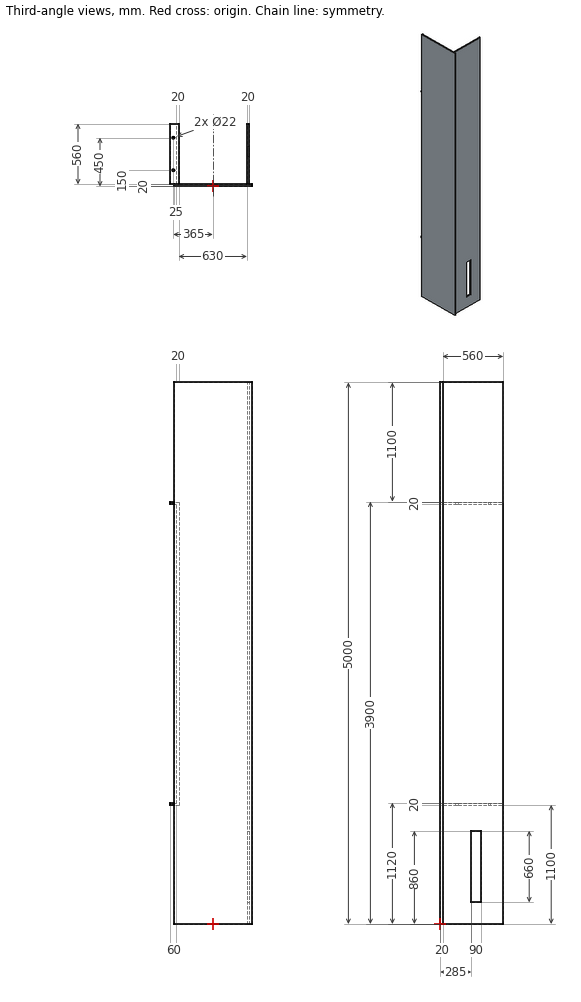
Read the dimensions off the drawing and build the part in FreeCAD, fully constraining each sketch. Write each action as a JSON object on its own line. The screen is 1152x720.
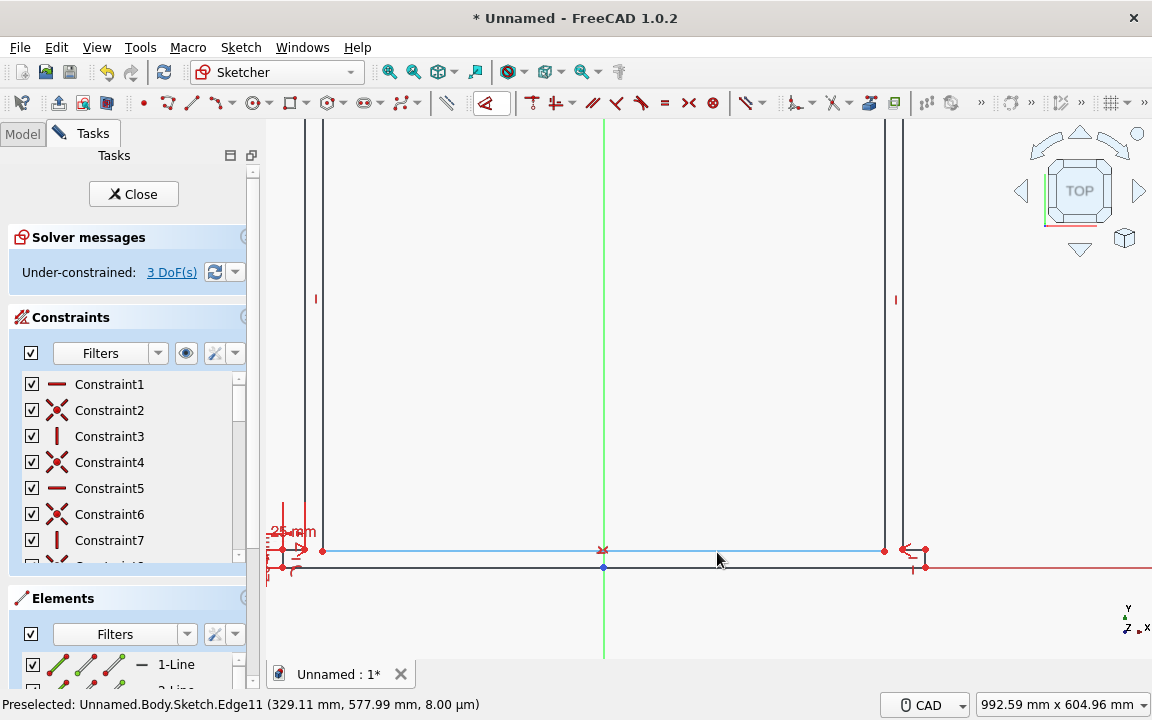
{"action": "left_click", "coordinate": [716, 551]}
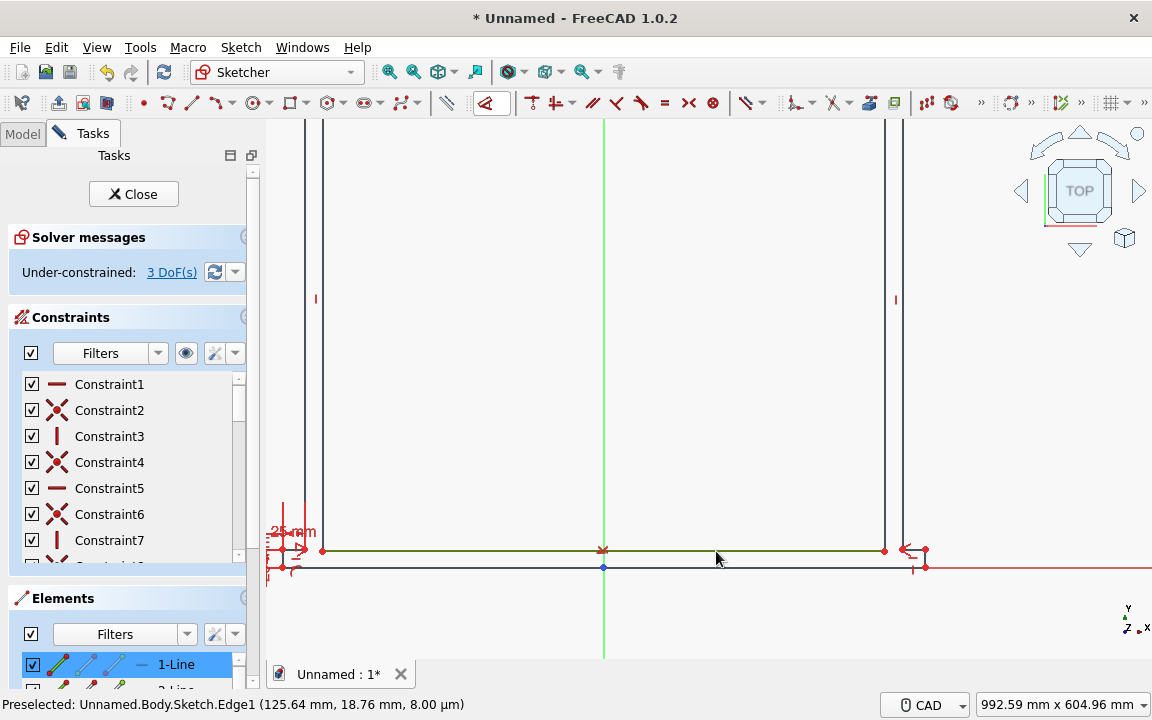
{"action": "left_click", "coordinate": [504, 104]}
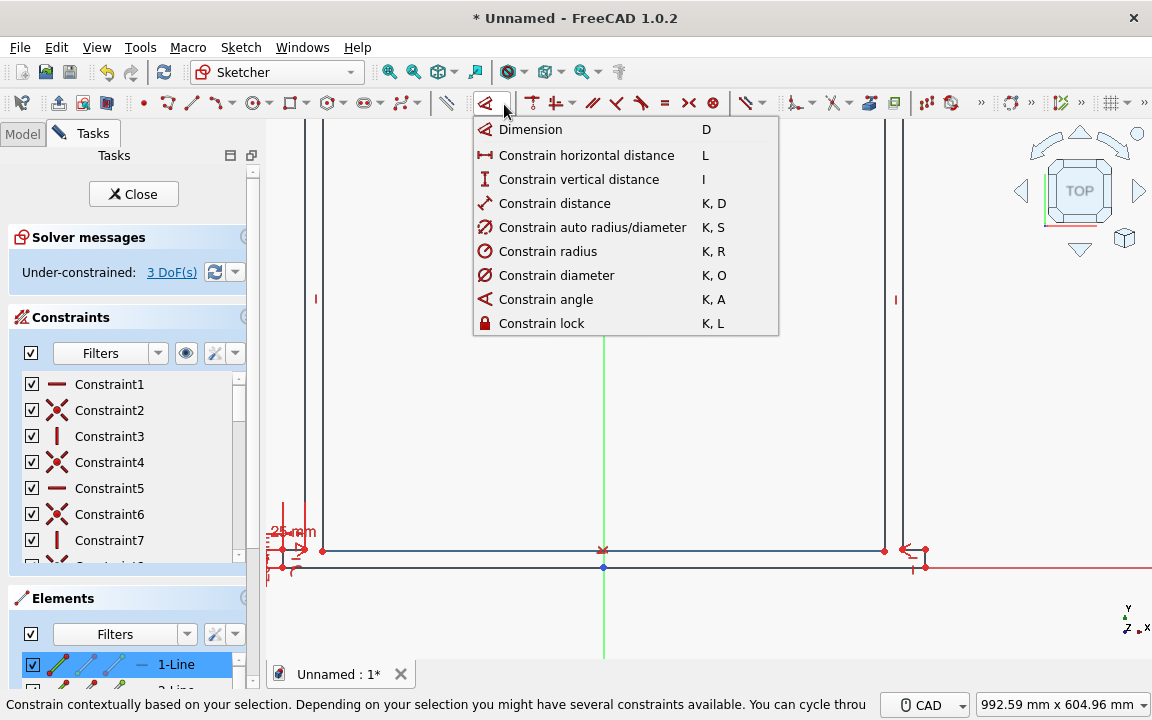
{"action": "left_click", "coordinate": [626, 155]}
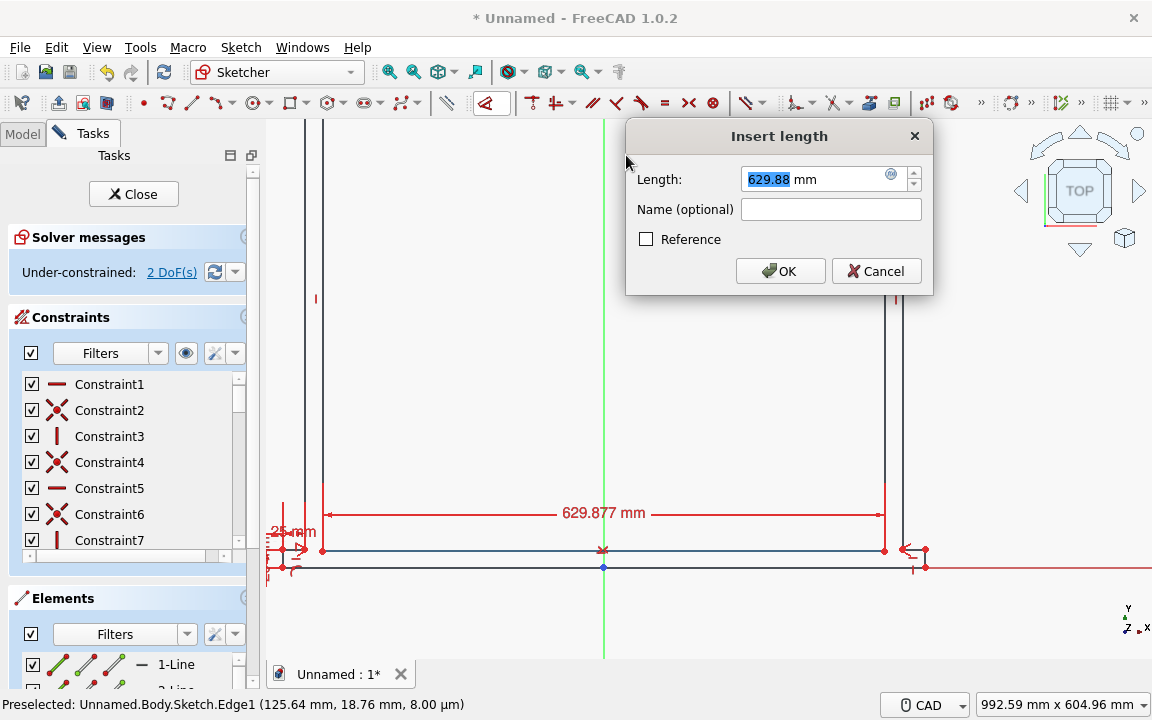
{"action": "type", "text": "630"}
{"action": "key", "text": "Return"}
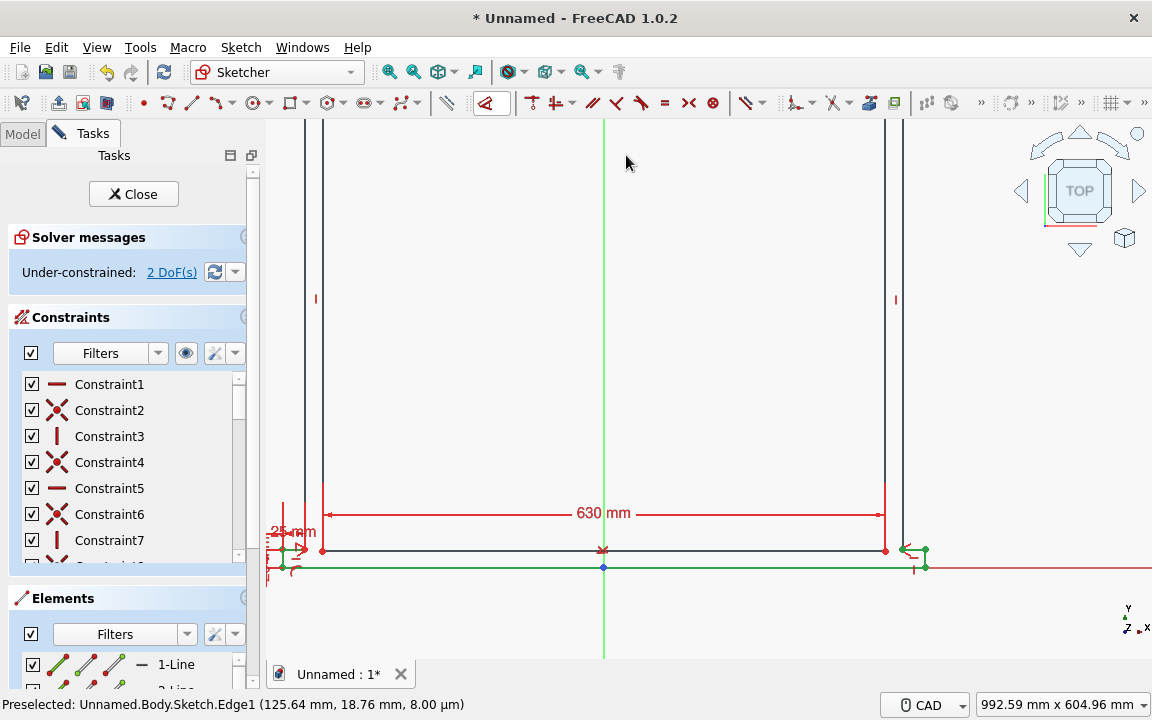
{"action": "left_click", "coordinate": [323, 401]}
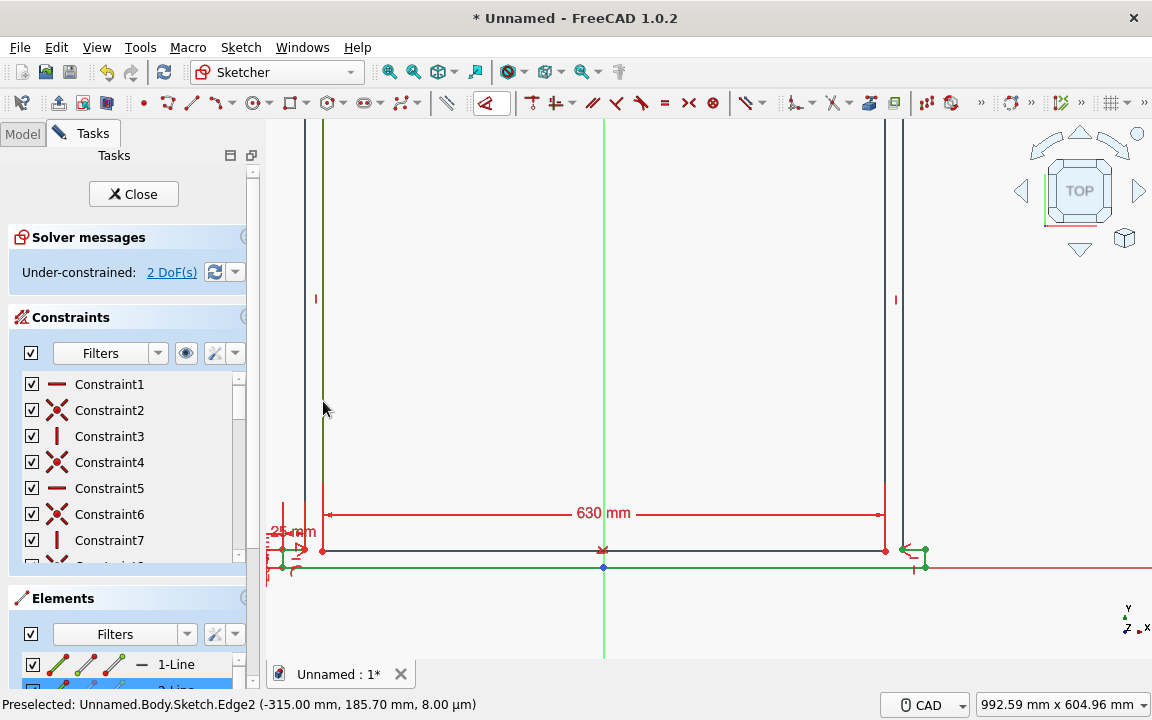
{"action": "left_click", "coordinate": [504, 104]}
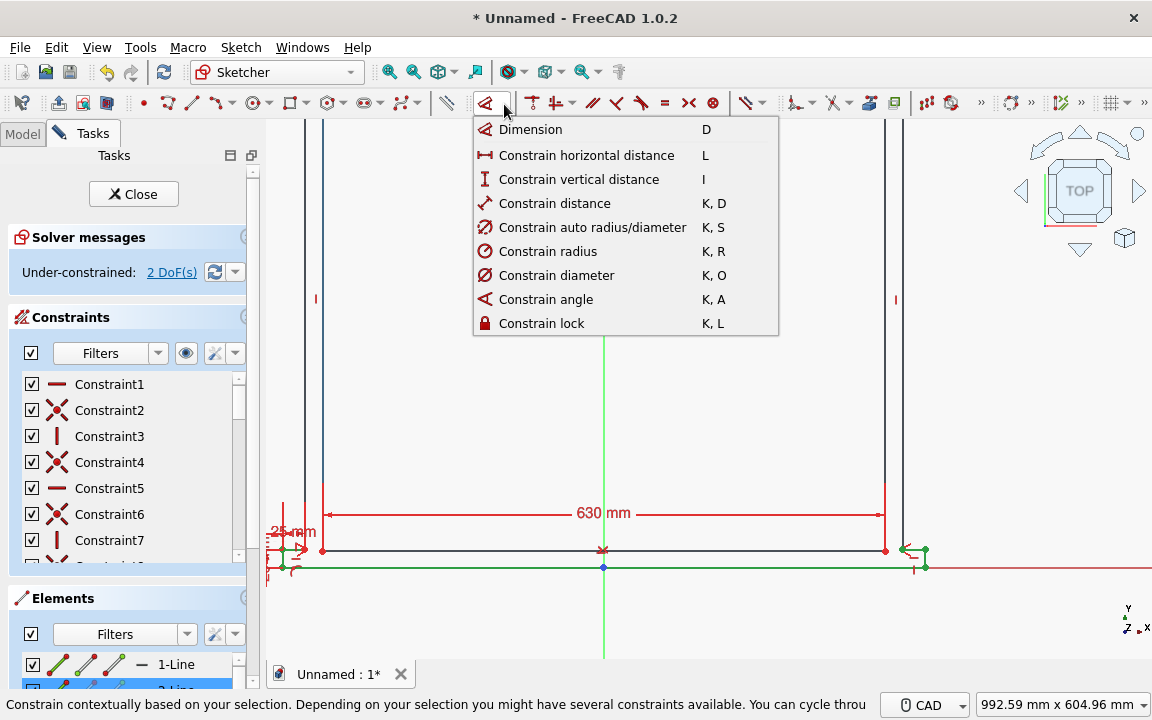
{"action": "left_click", "coordinate": [626, 179]}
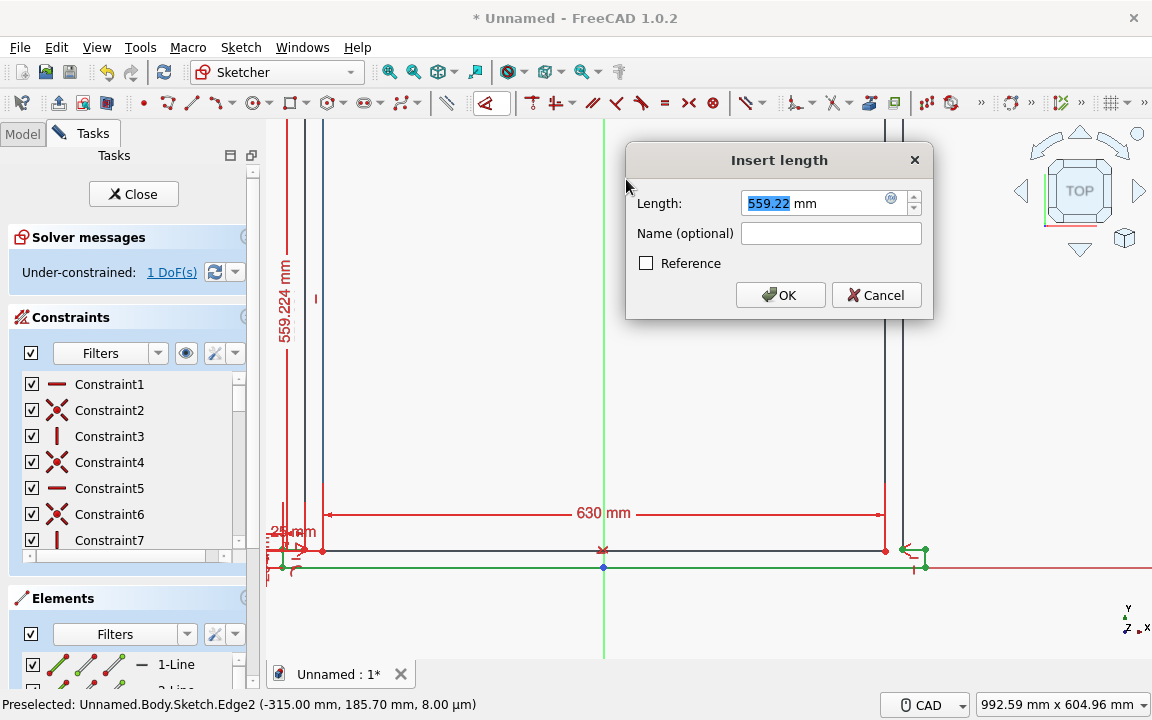
{"action": "type", "text": "560"}
{"action": "key", "text": "Return"}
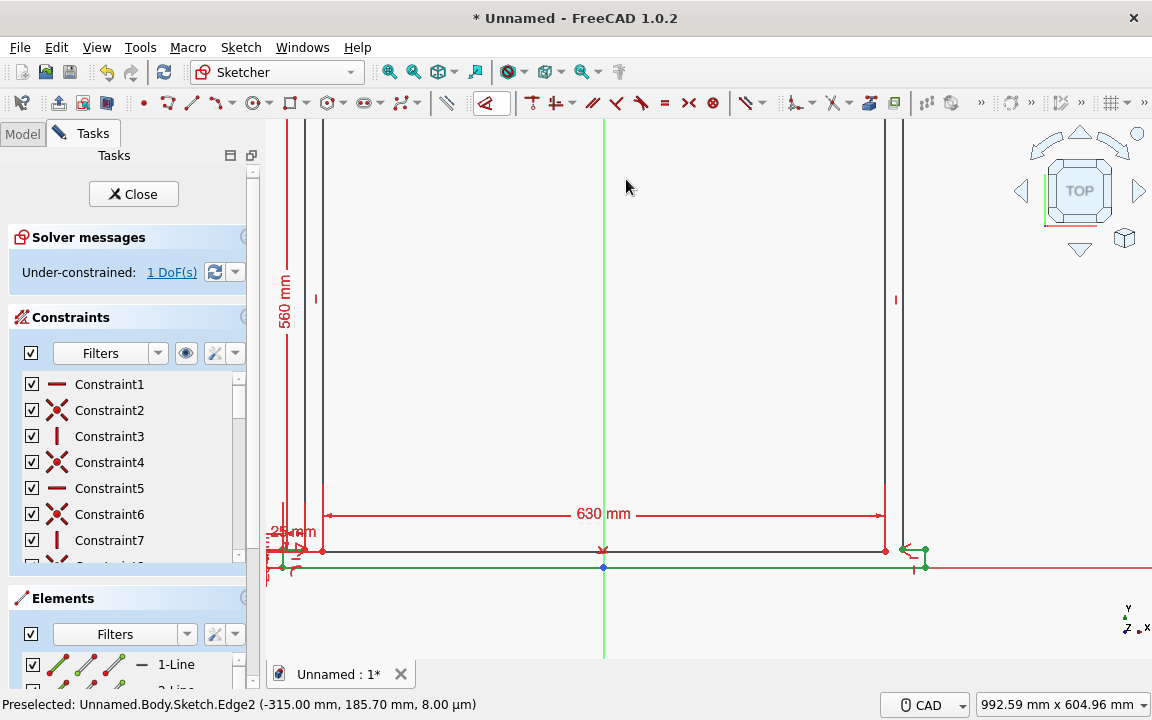
{"action": "left_click", "coordinate": [305, 201]}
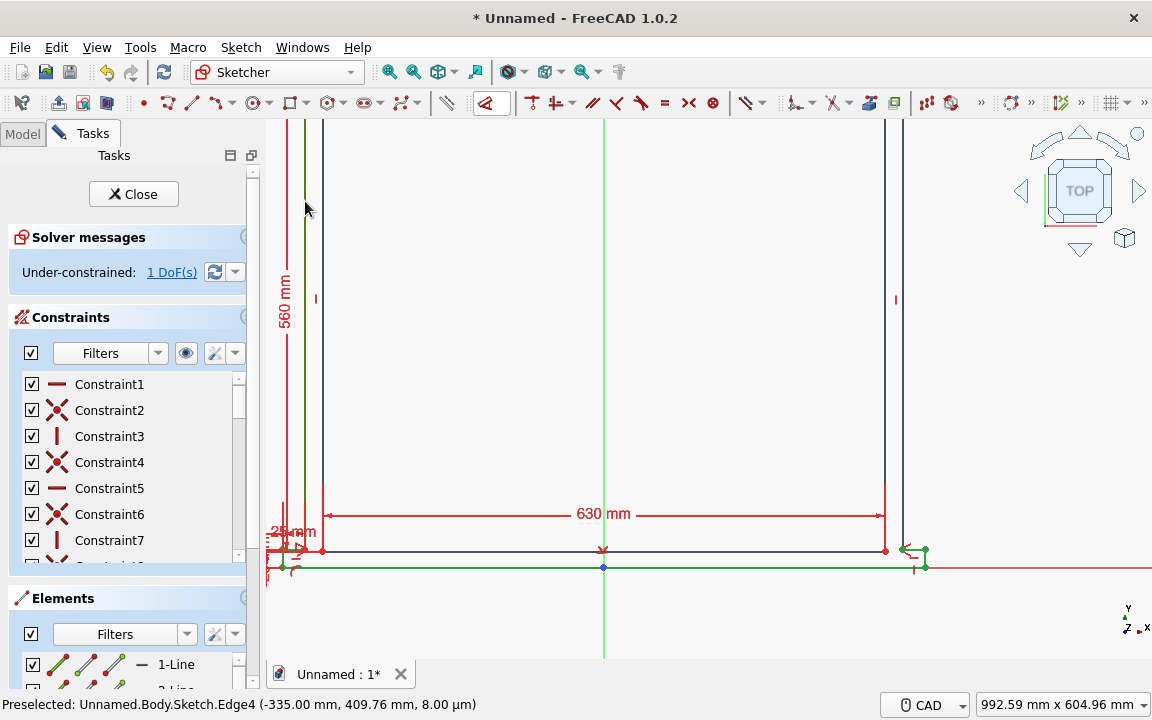
{"action": "key", "text": "i"}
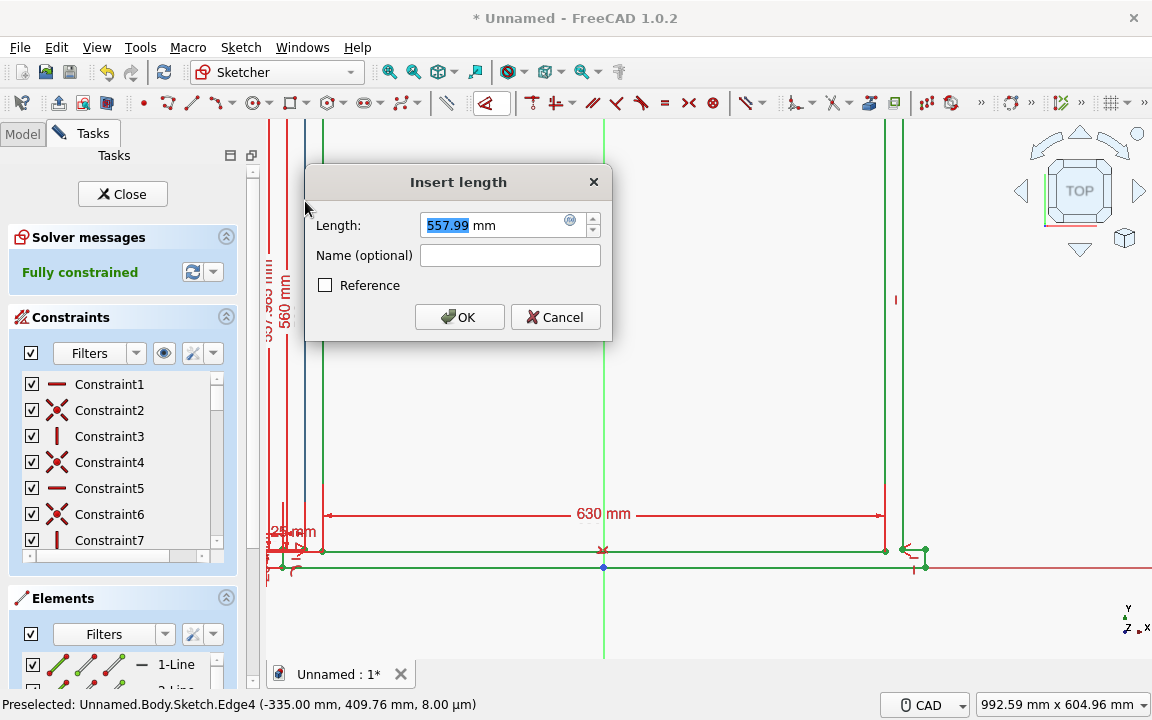
{"action": "type", "text": "560"}
{"action": "key", "text": "Return"}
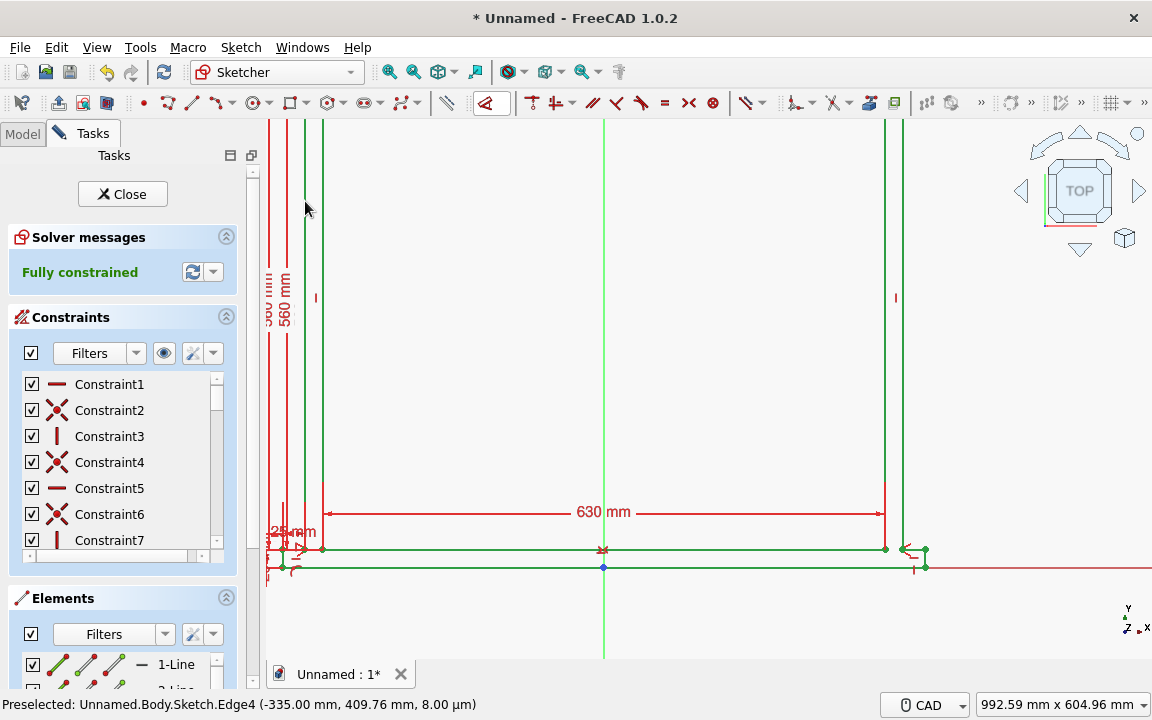
{"action": "left_click", "coordinate": [123, 194]}